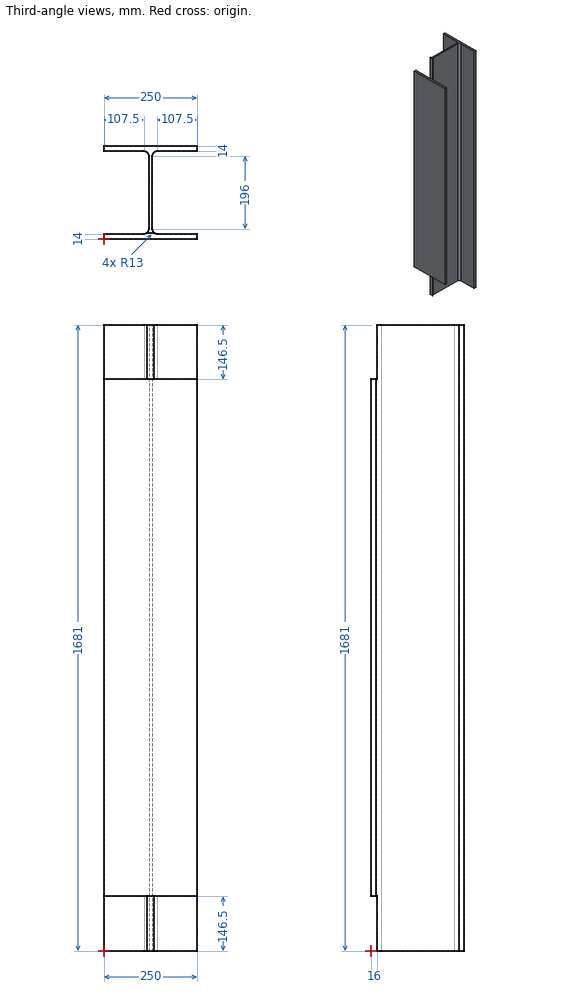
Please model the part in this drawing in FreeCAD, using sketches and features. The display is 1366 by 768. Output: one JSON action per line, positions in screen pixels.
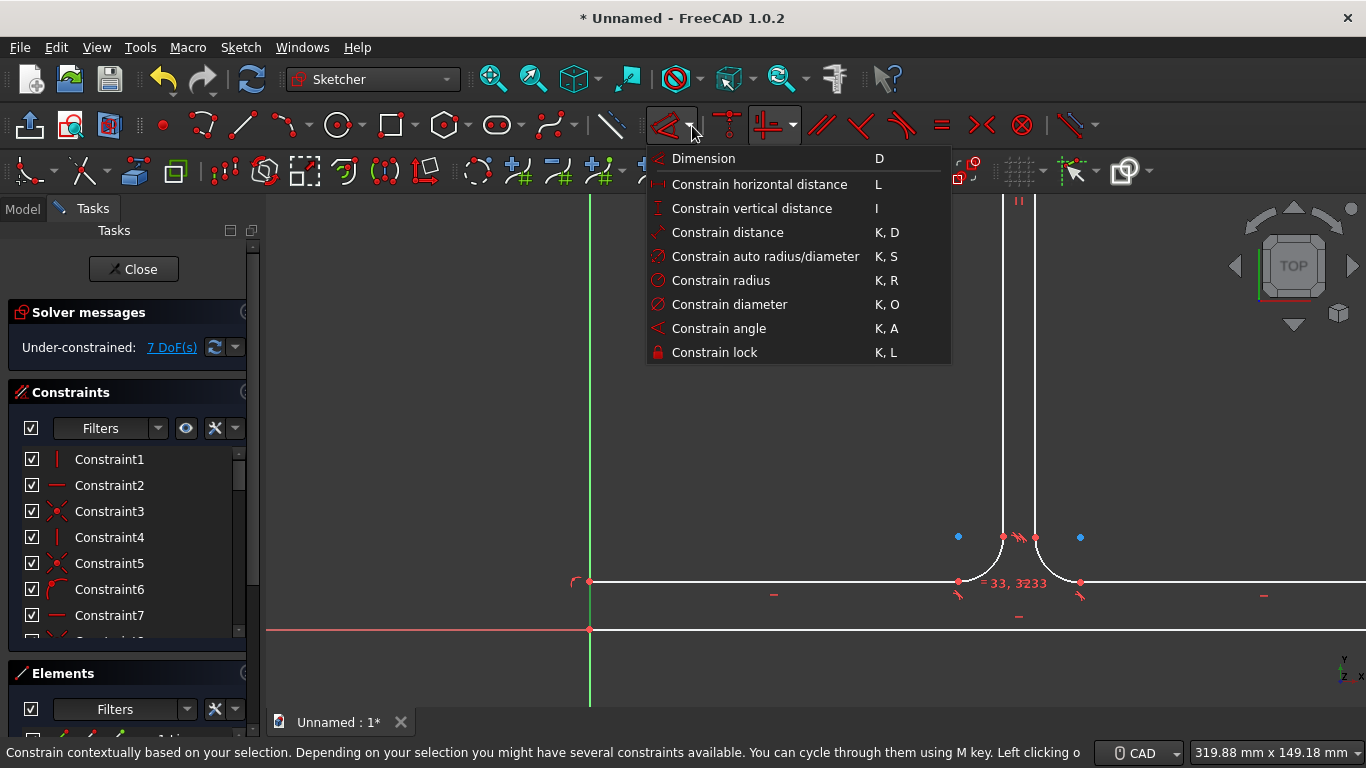
{"action": "left_click", "coordinate": [799, 208]}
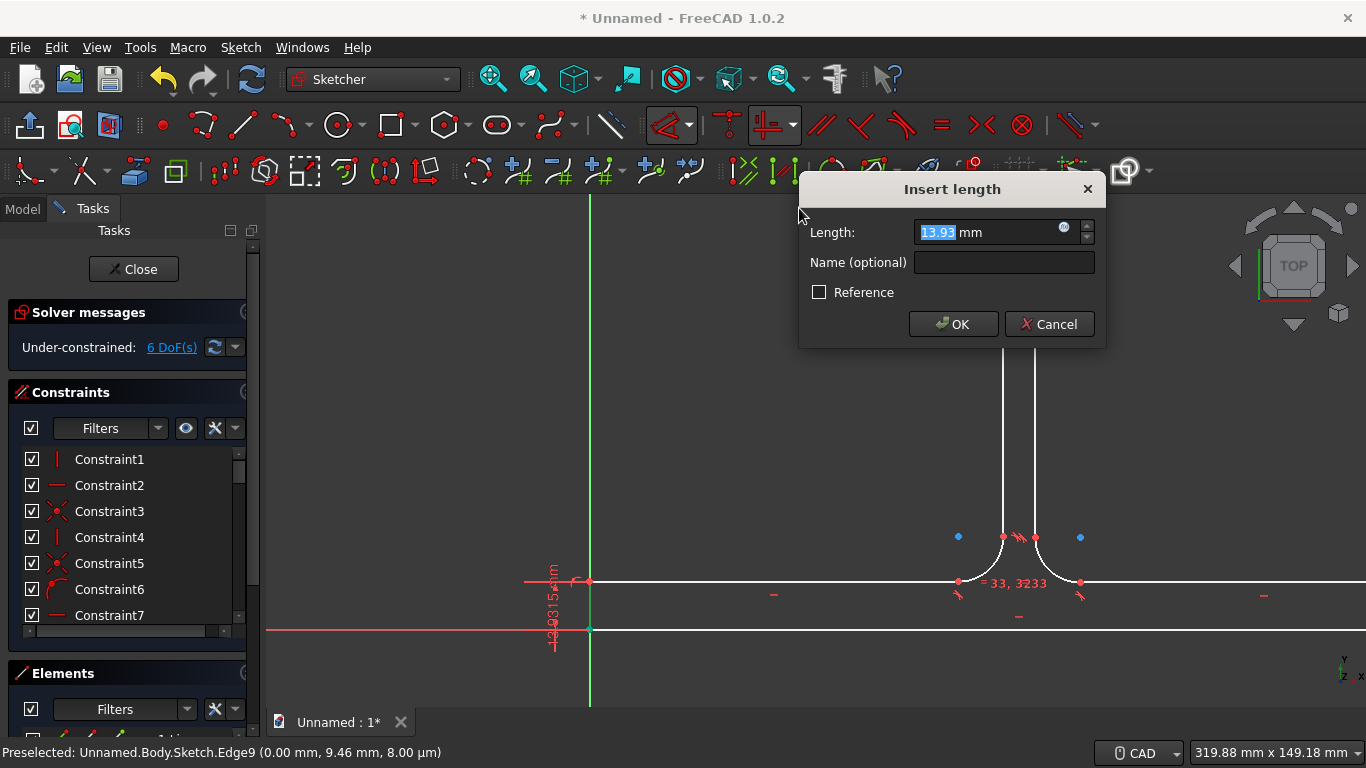
{"action": "type", "text": "14"}
{"action": "key", "text": "Return"}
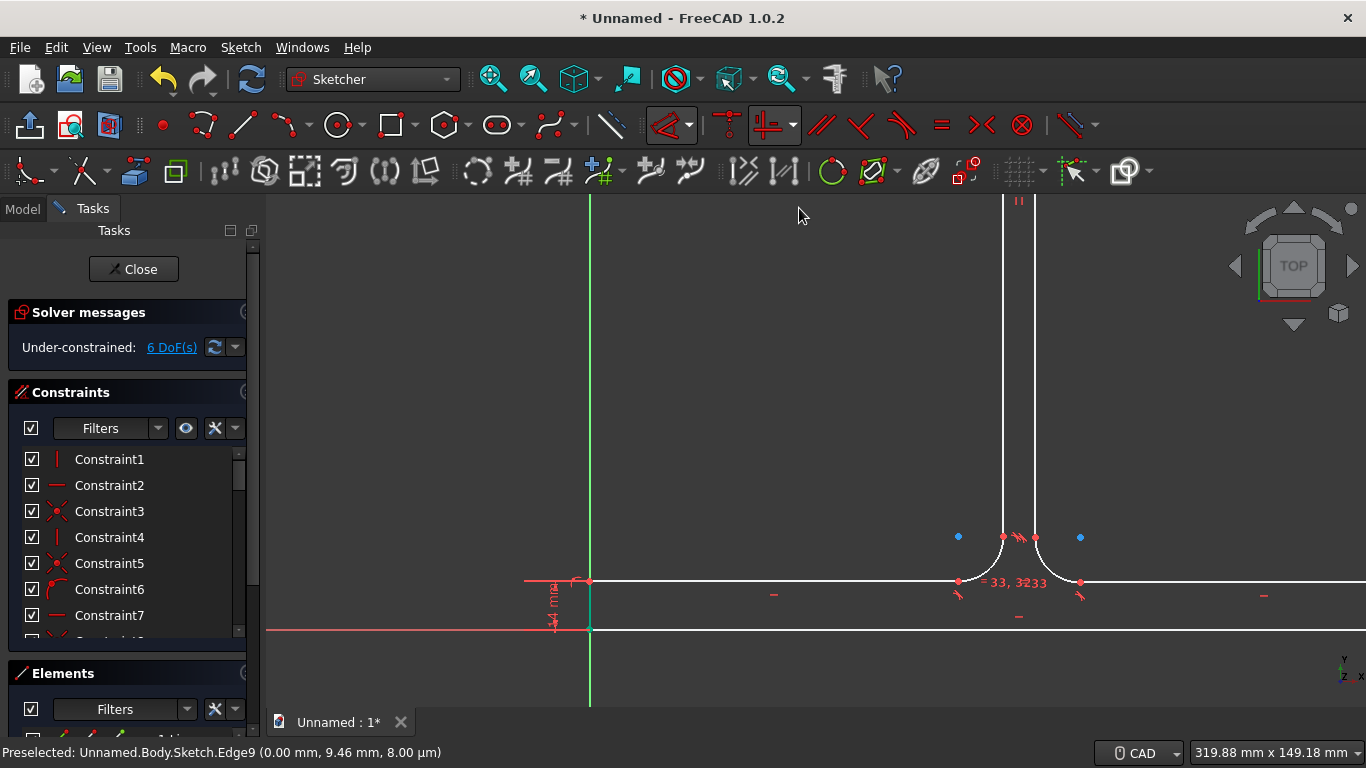
{"action": "scroll", "coordinate": [589, 596], "scroll_direction": "down", "scroll_amount": 5}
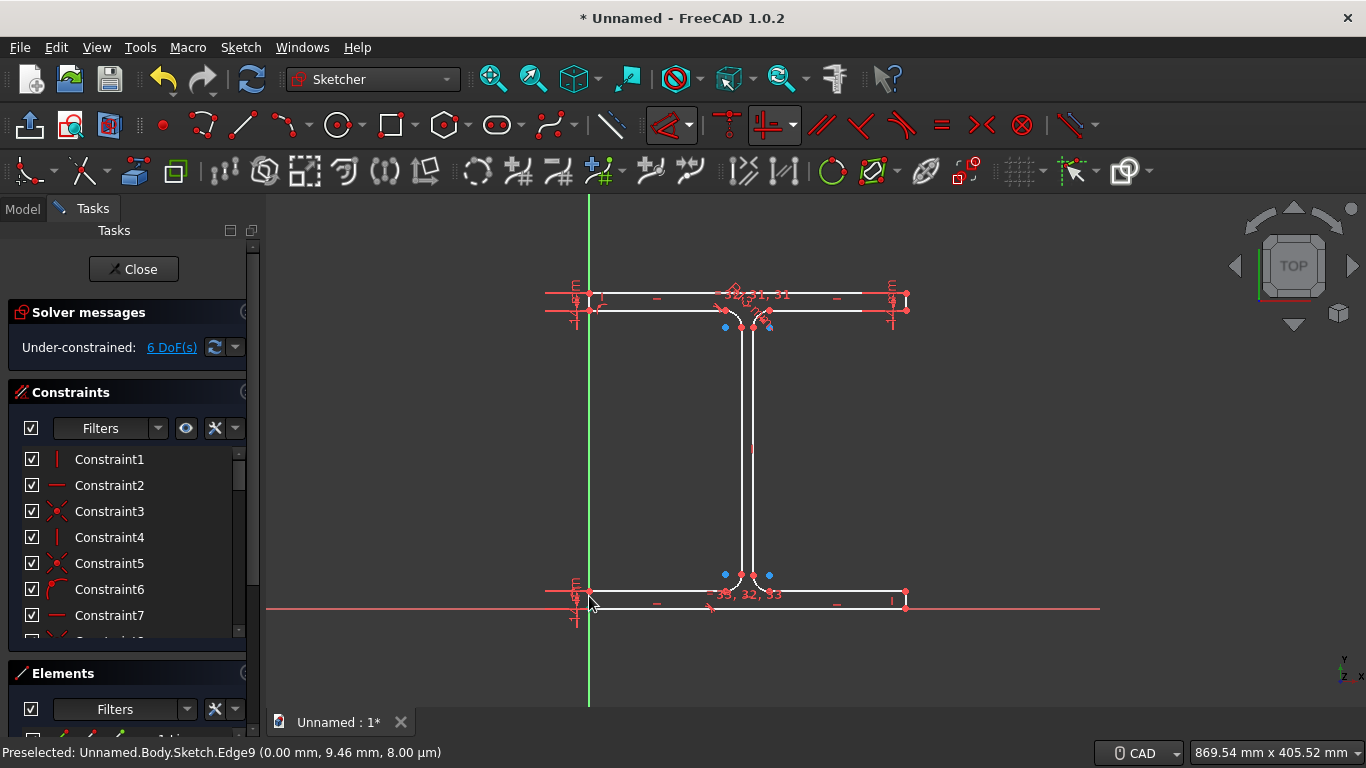
{"action": "scroll", "coordinate": [906, 604], "scroll_direction": "up", "scroll_amount": 5}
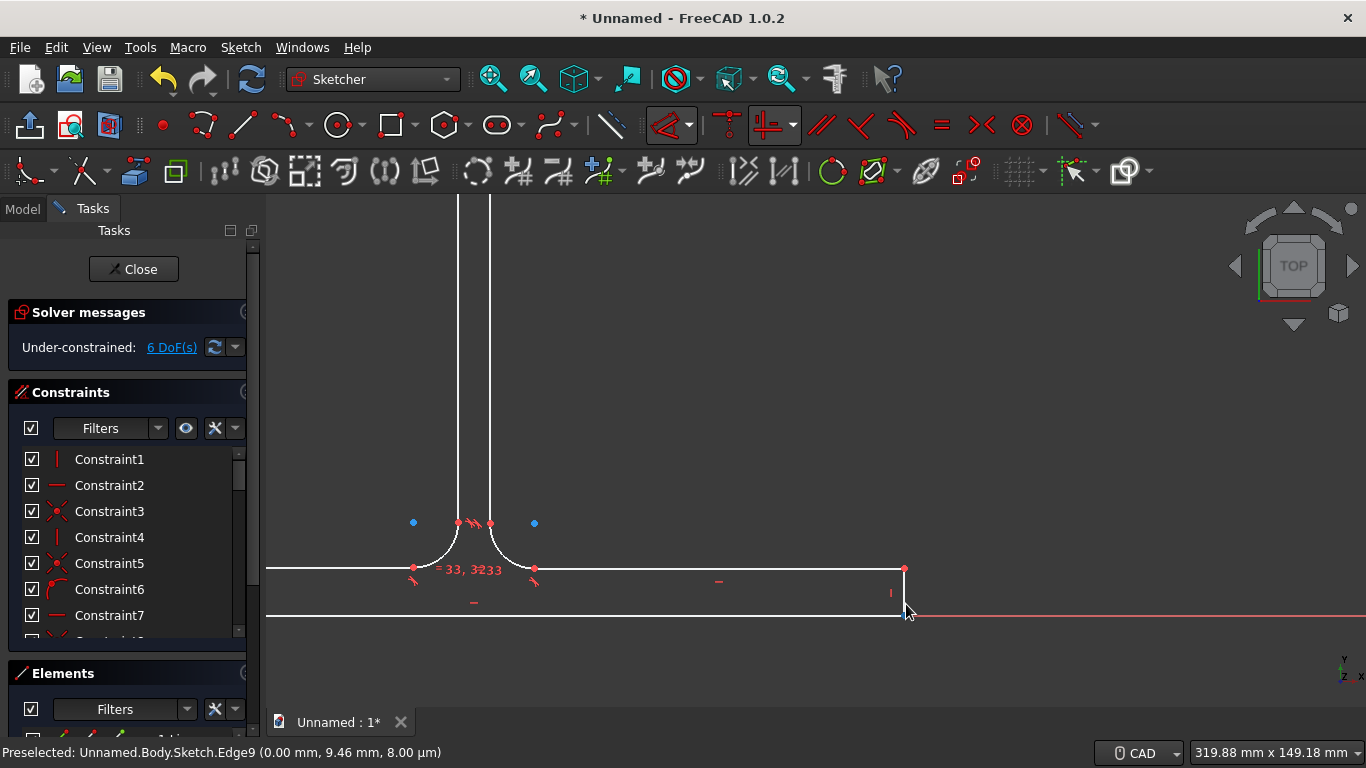
{"action": "left_click", "coordinate": [904, 602]}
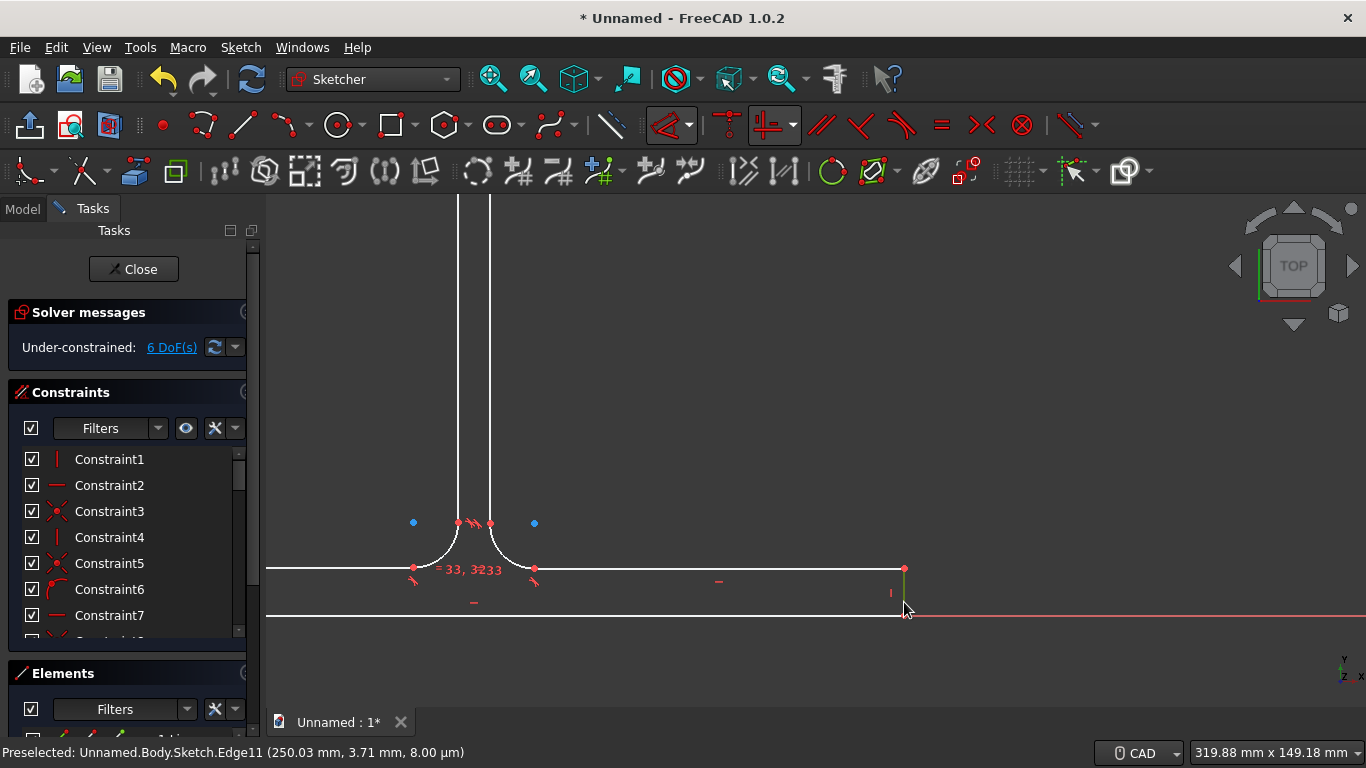
{"action": "left_click", "coordinate": [692, 126]}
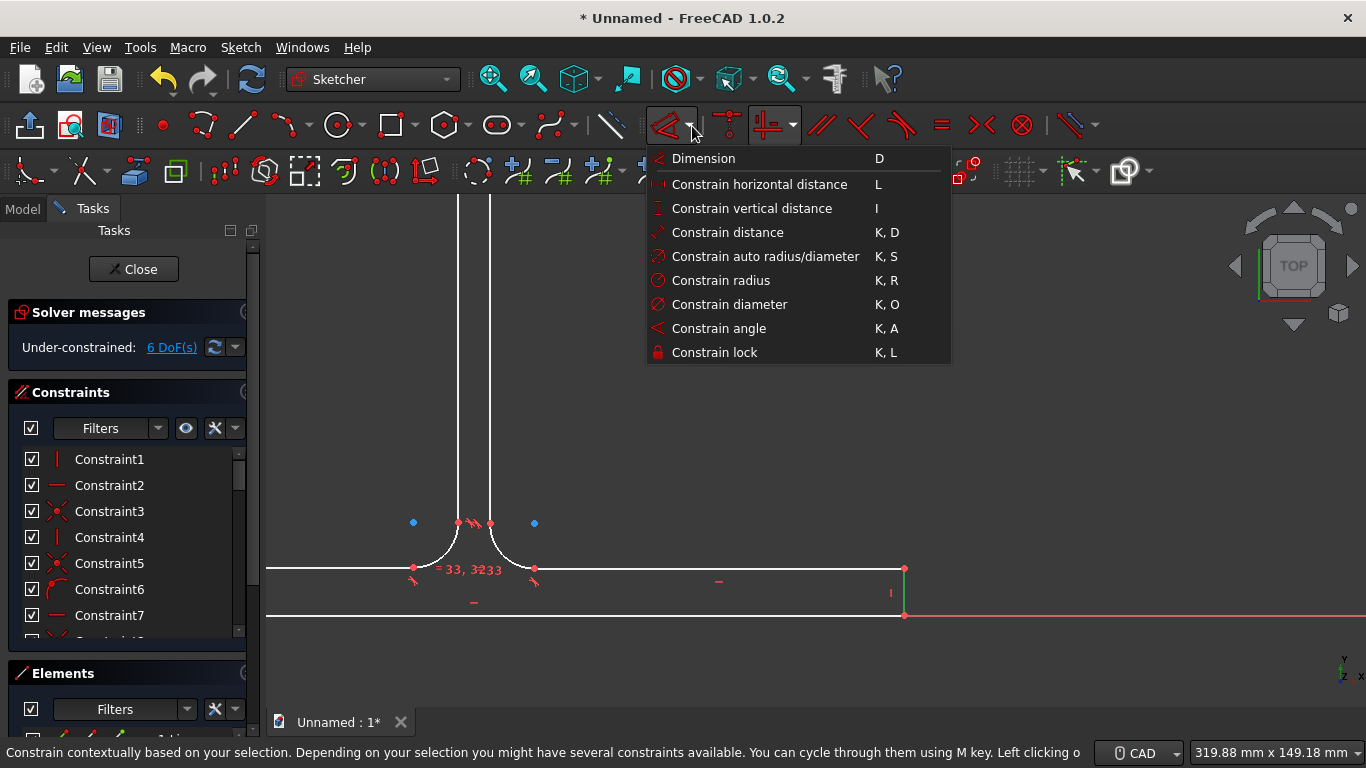
{"action": "left_click", "coordinate": [799, 208]}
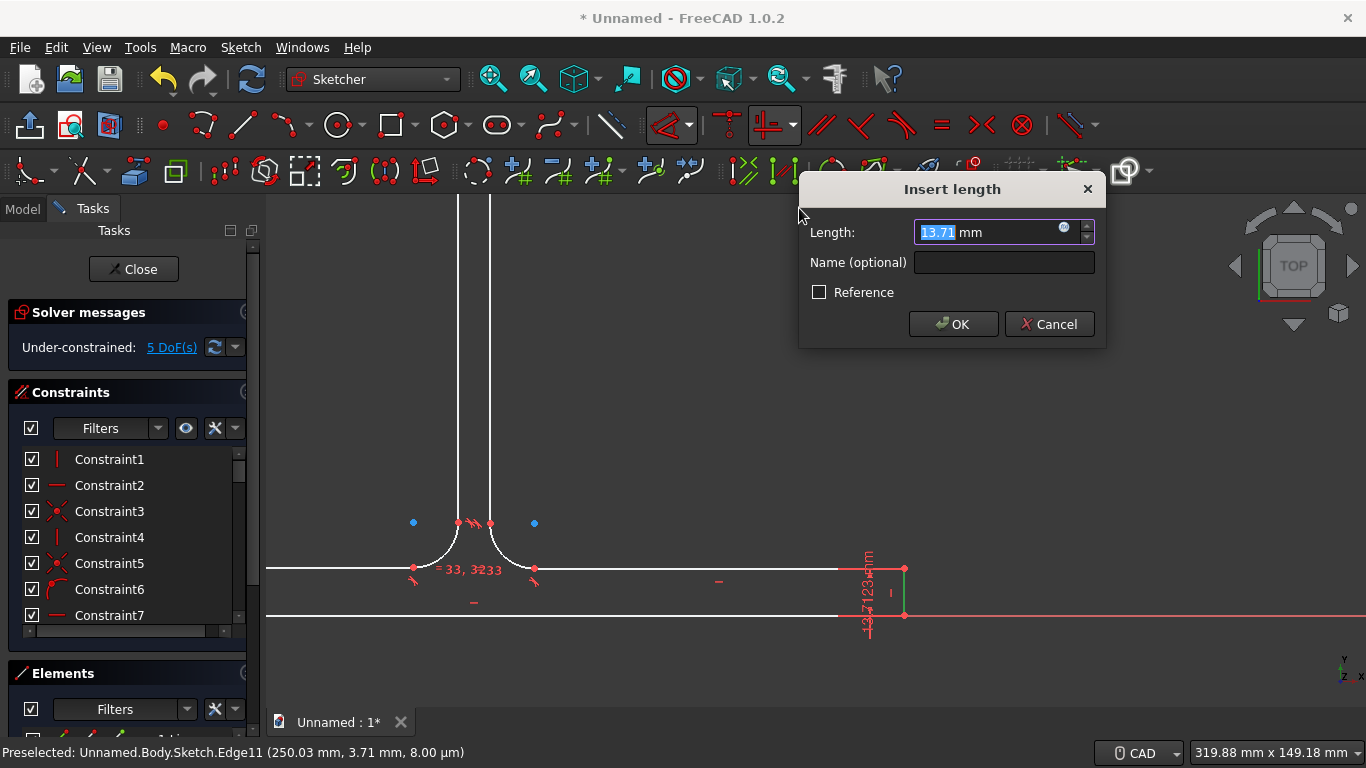
{"action": "type", "text": "14"}
{"action": "key", "text": "Return"}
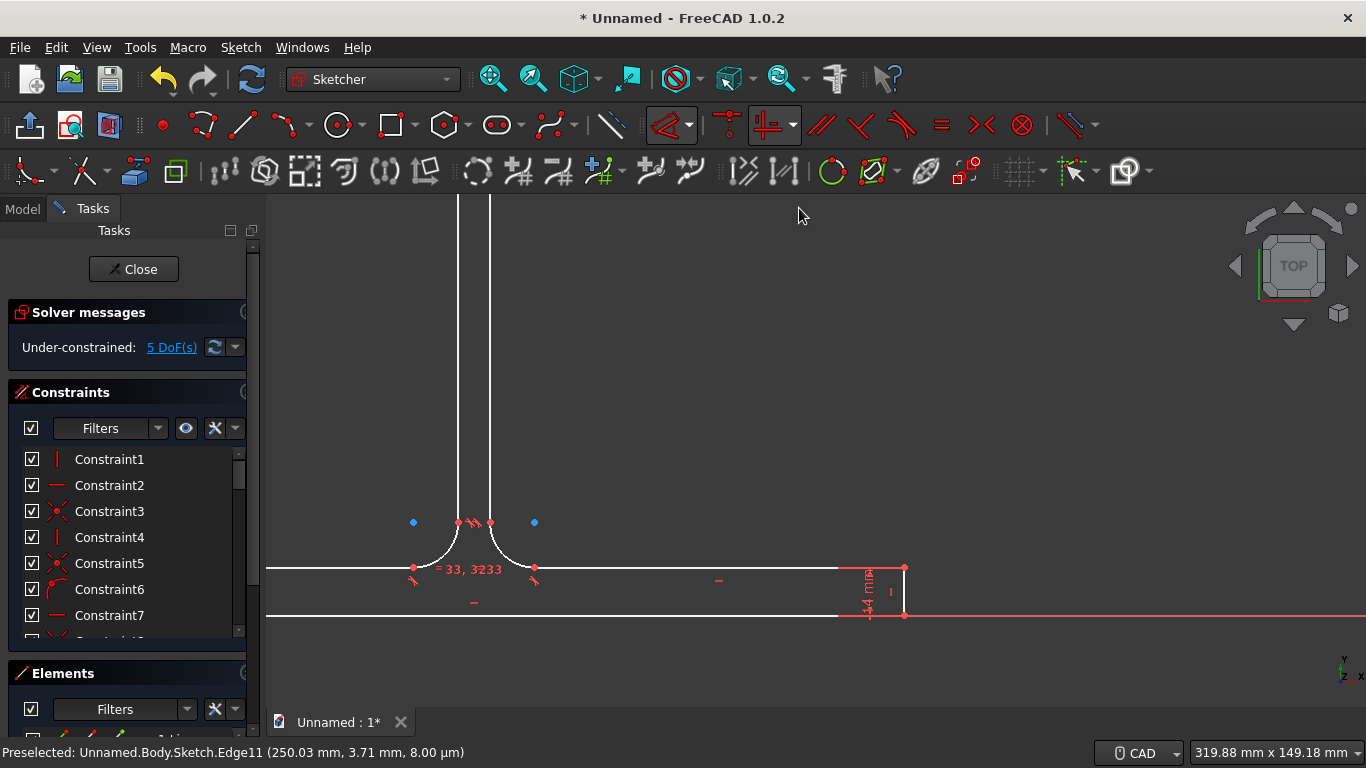
{"action": "left_click", "coordinate": [490, 321]}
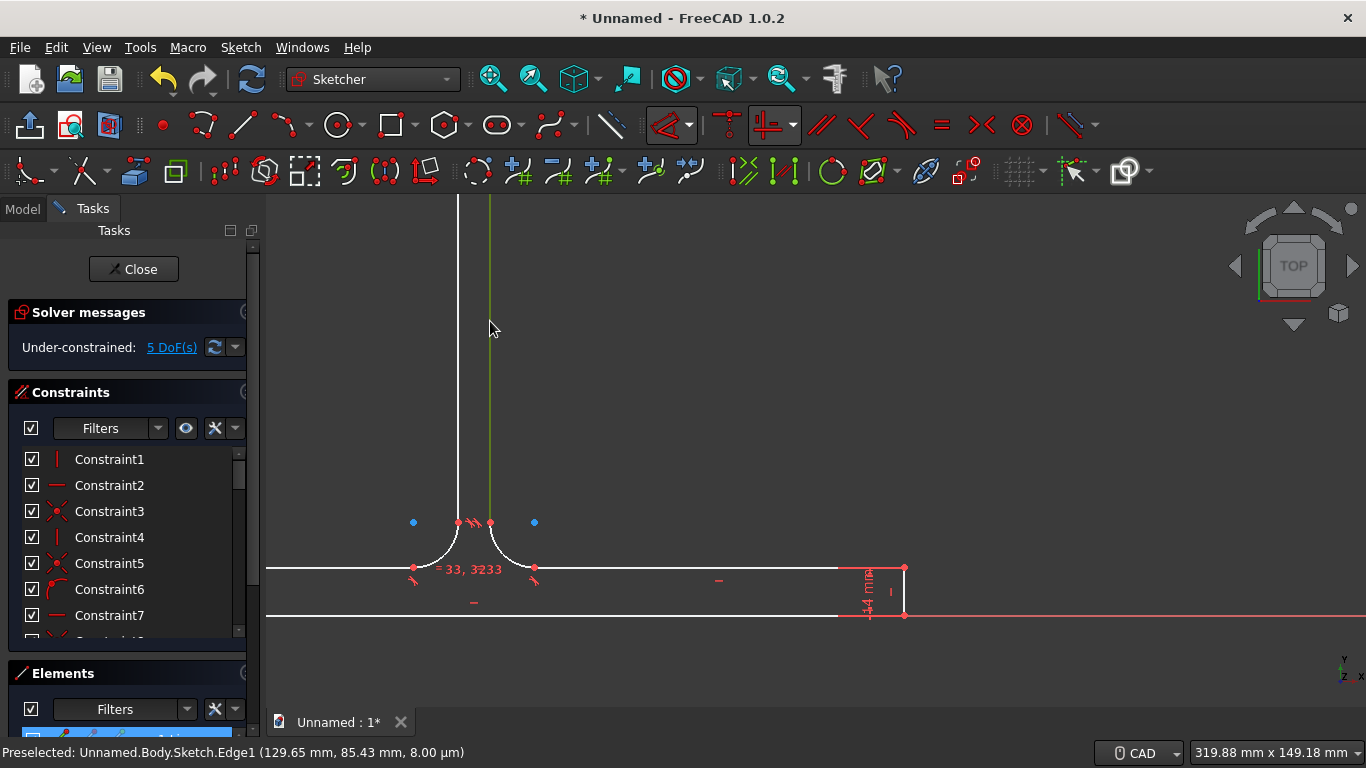
{"action": "key", "text": "i"}